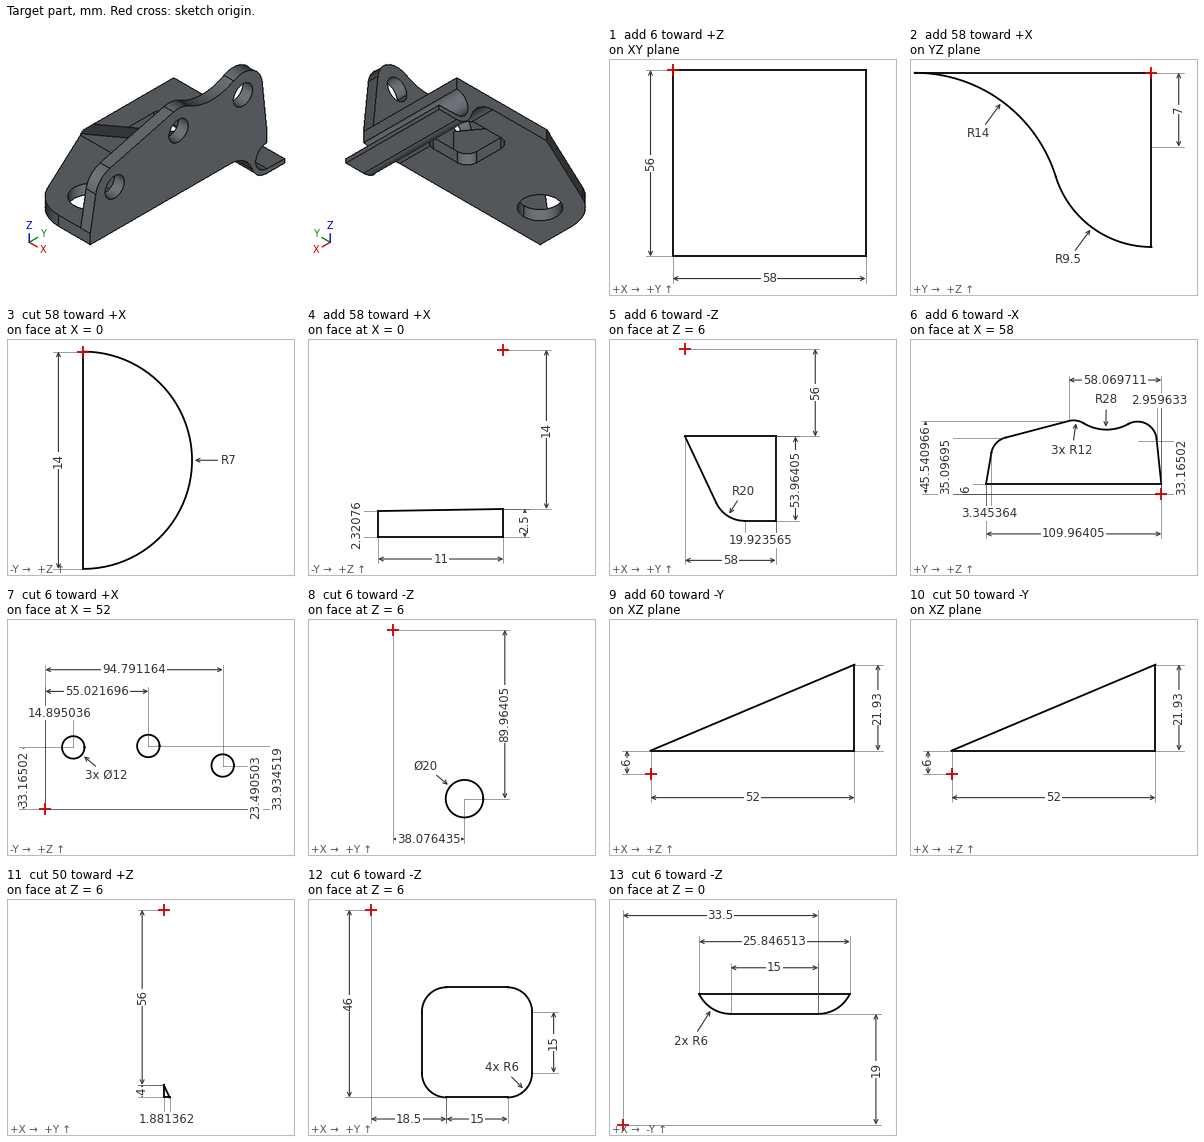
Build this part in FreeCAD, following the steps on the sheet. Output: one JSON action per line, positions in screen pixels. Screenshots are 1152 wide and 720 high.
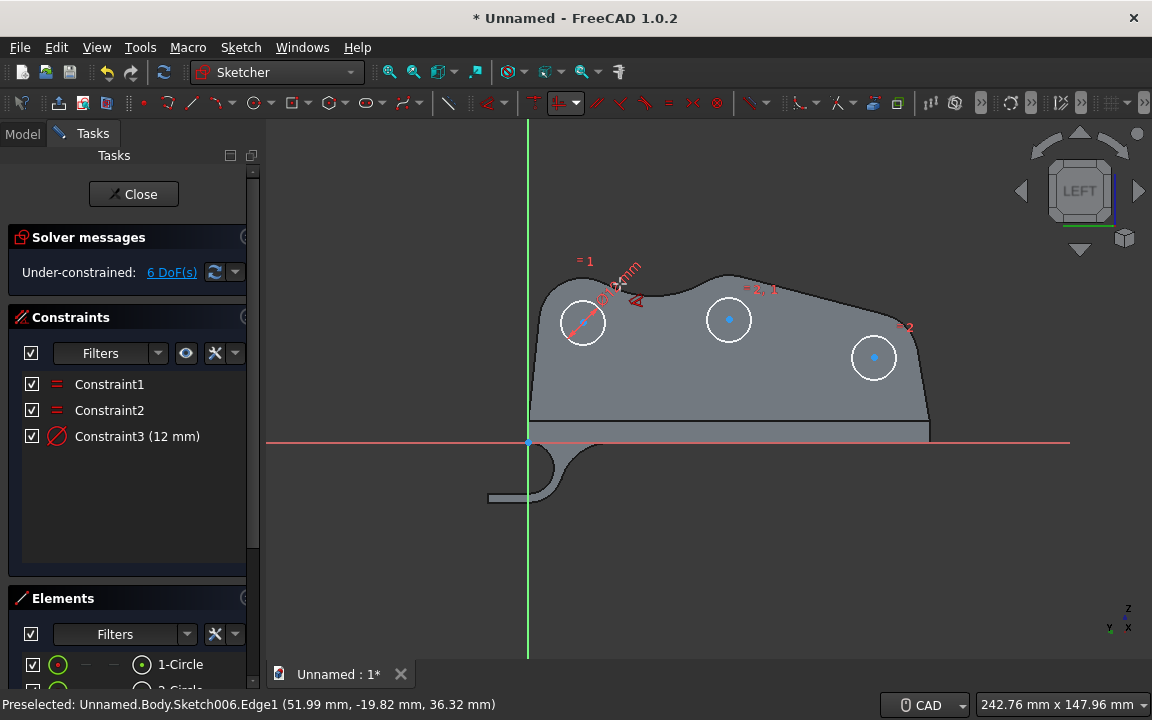
{"action": "left_click", "coordinate": [583, 323]}
{"action": "left_click", "coordinate": [494, 383]}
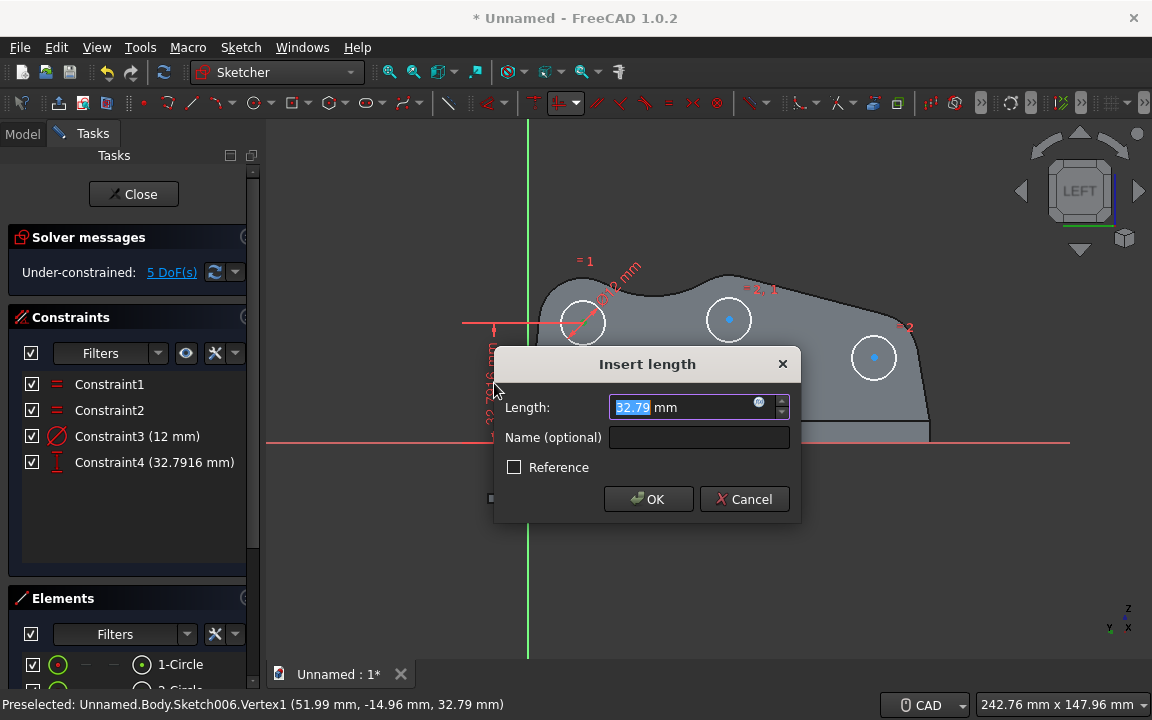
{"action": "type", "text": "33.16502"}
{"action": "key", "text": "Return"}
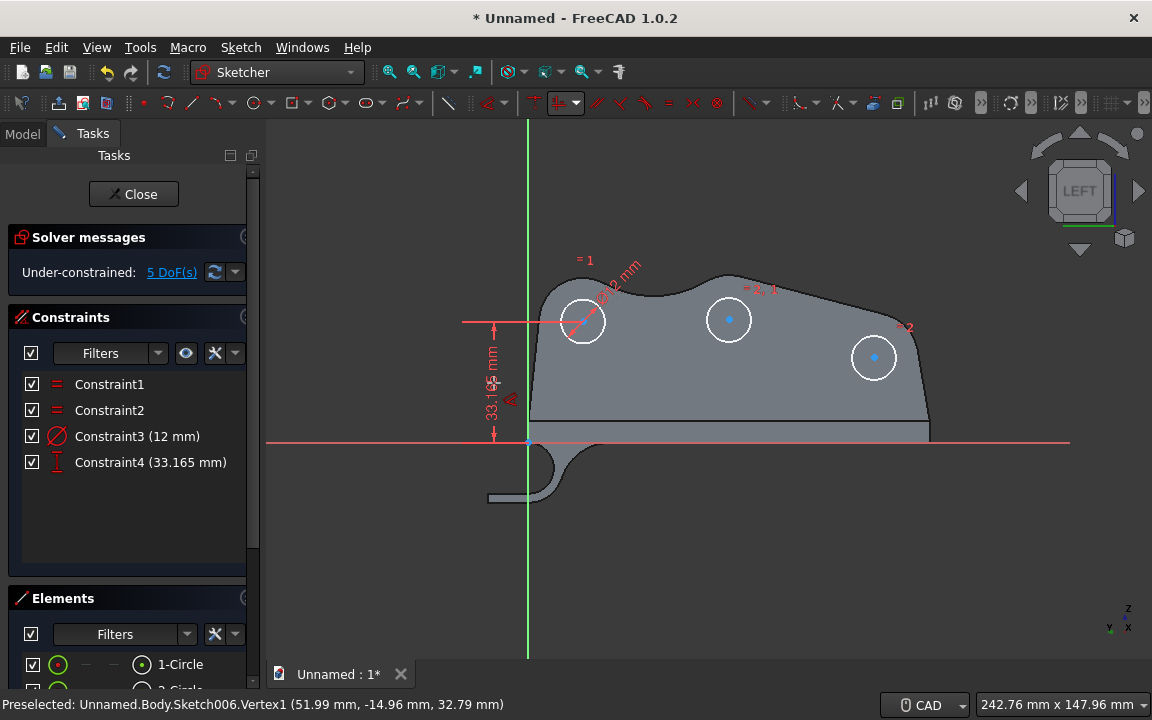
{"action": "left_click", "coordinate": [583, 322]}
{"action": "left_click", "coordinate": [556, 477]}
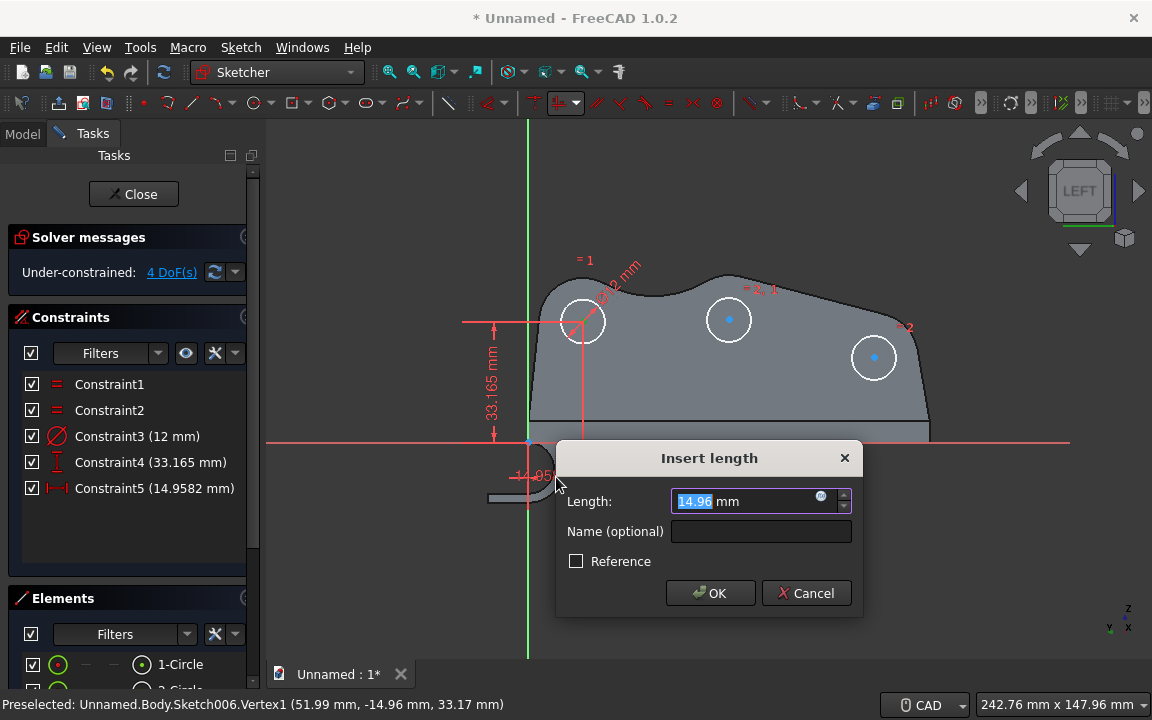
{"action": "type", "text": "14.895036"}
{"action": "key", "text": "Return"}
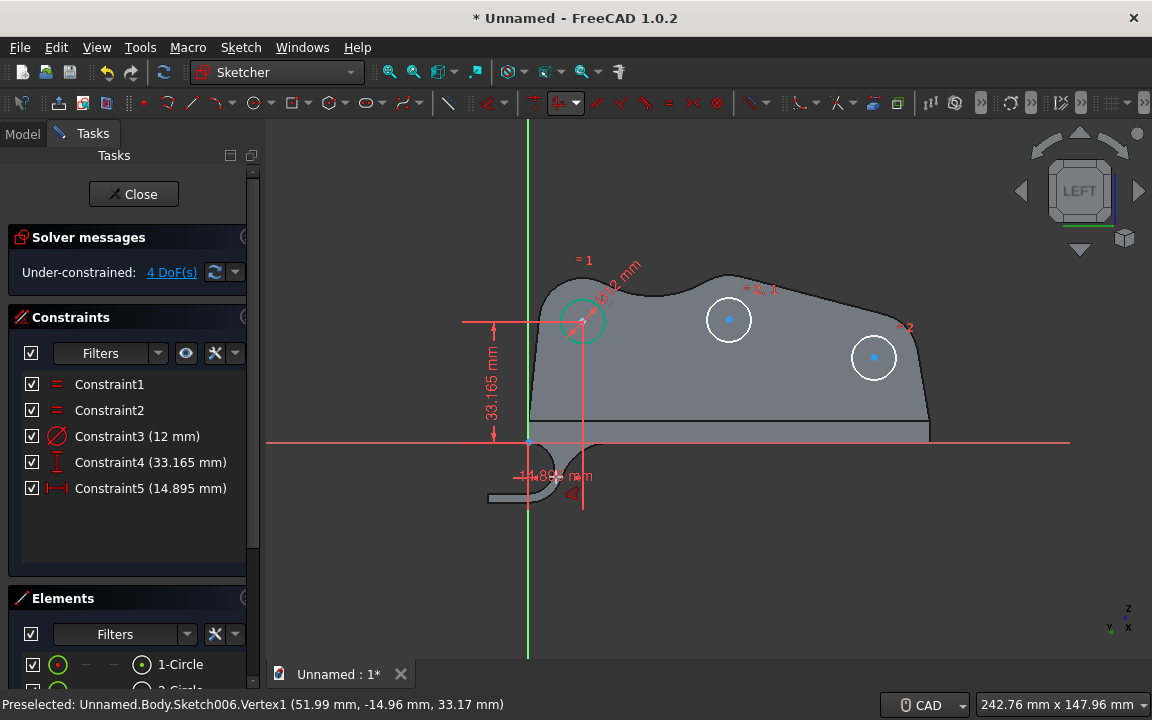
{"action": "left_click", "coordinate": [729, 320]}
{"action": "left_click", "coordinate": [629, 477]}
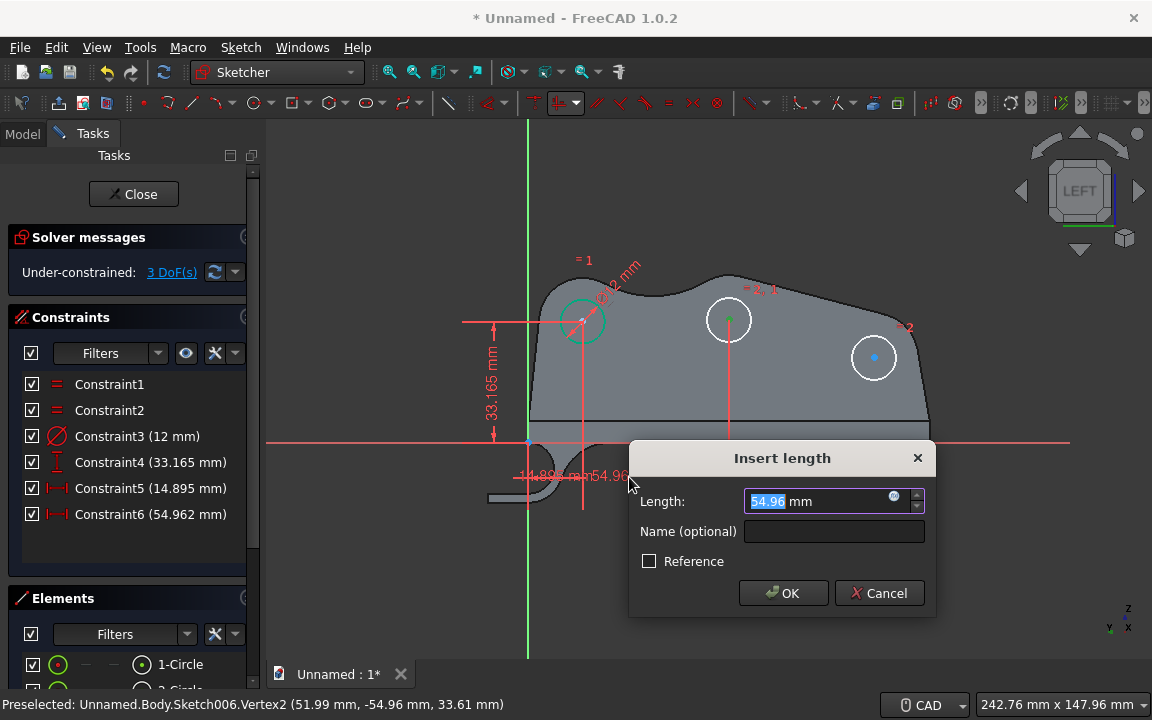
{"action": "type", "text": "55.021696"}
{"action": "key", "text": "Return"}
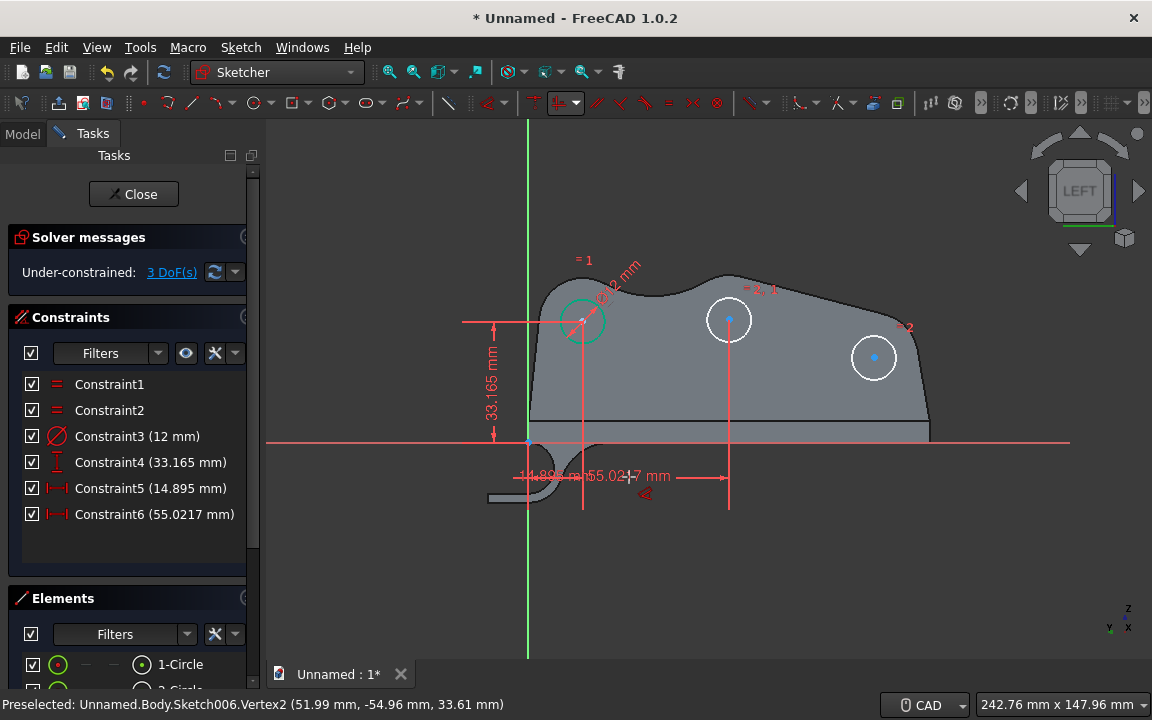
{"action": "left_click", "coordinate": [729, 320]}
{"action": "left_click", "coordinate": [494, 353]}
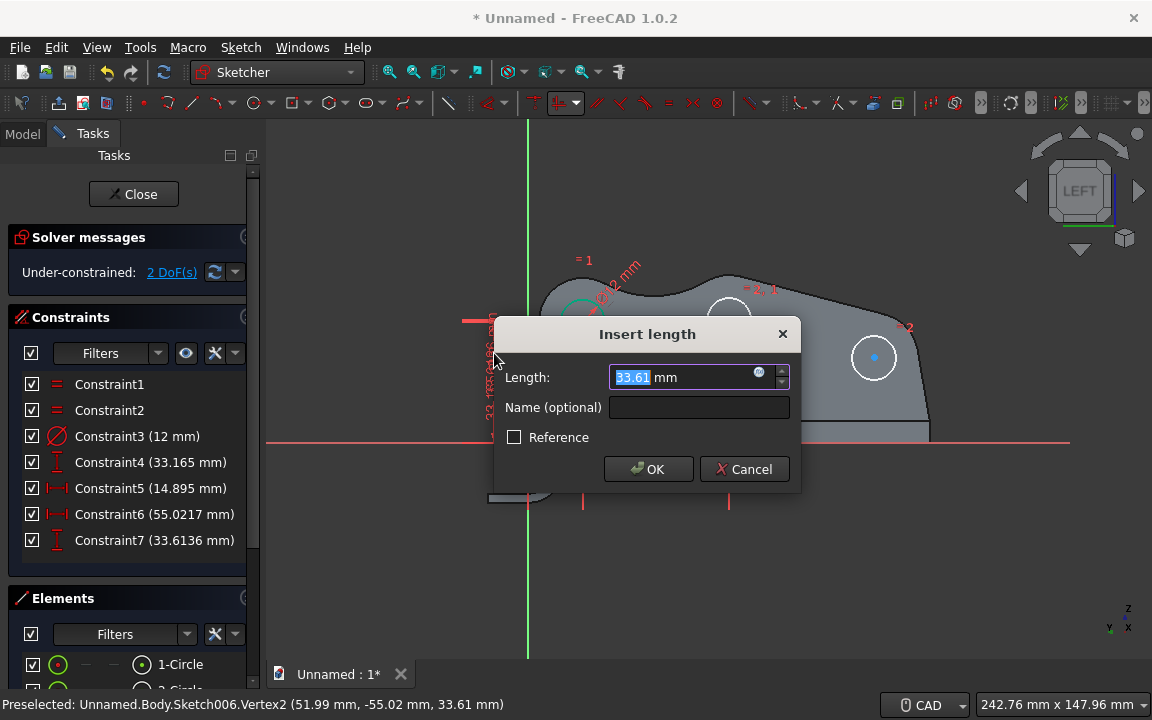
{"action": "type", "text": "33.934519"}
{"action": "key", "text": "Return"}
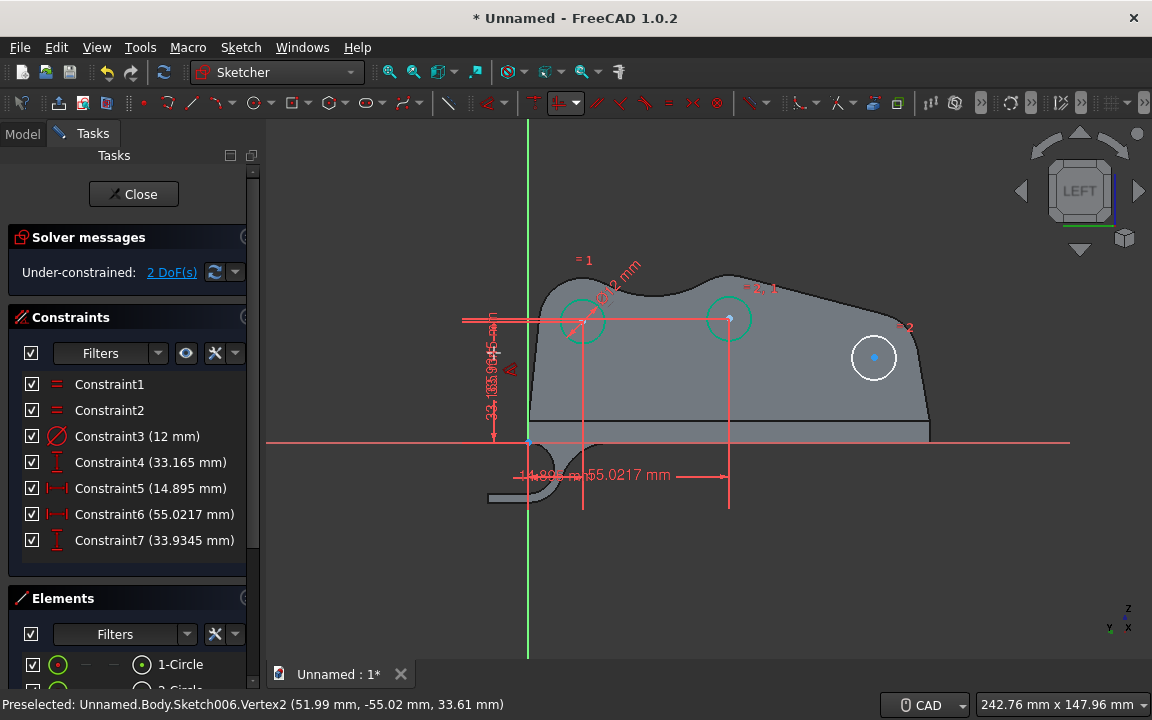
{"action": "left_click", "coordinate": [874, 358]}
{"action": "left_click", "coordinate": [701, 477]}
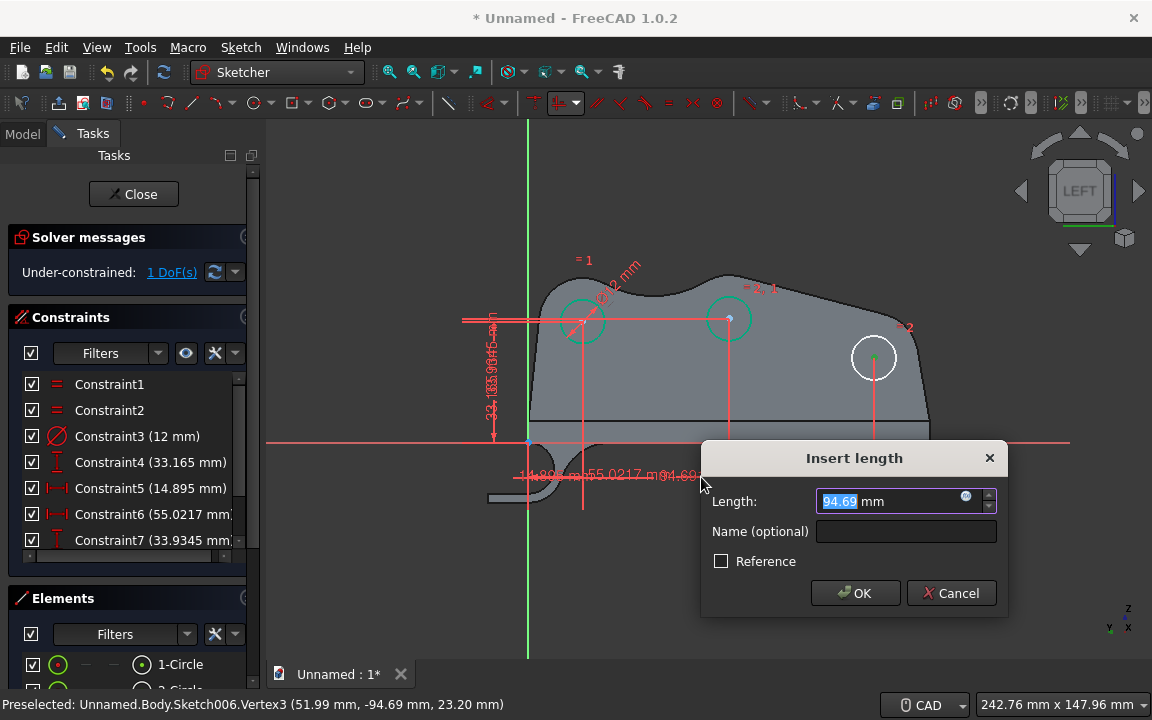
{"action": "type", "text": "94.791164"}
{"action": "key", "text": "Return"}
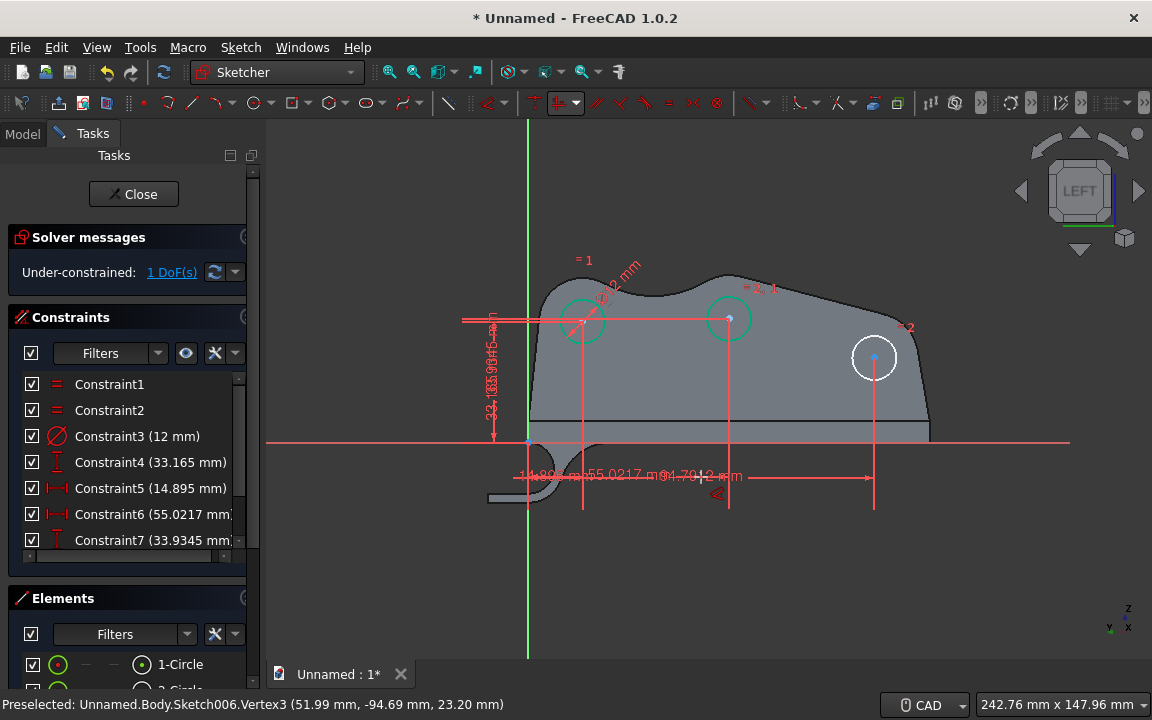
{"action": "left_click", "coordinate": [874, 358]}
{"action": "left_click", "coordinate": [494, 420]}